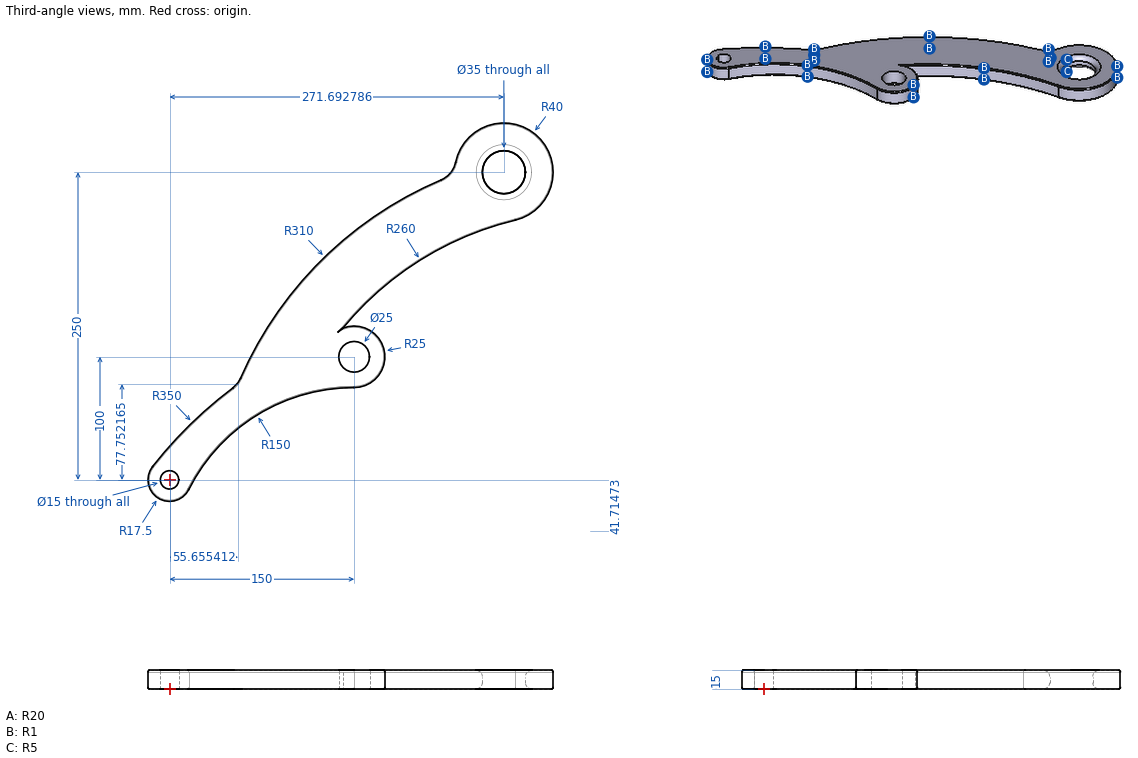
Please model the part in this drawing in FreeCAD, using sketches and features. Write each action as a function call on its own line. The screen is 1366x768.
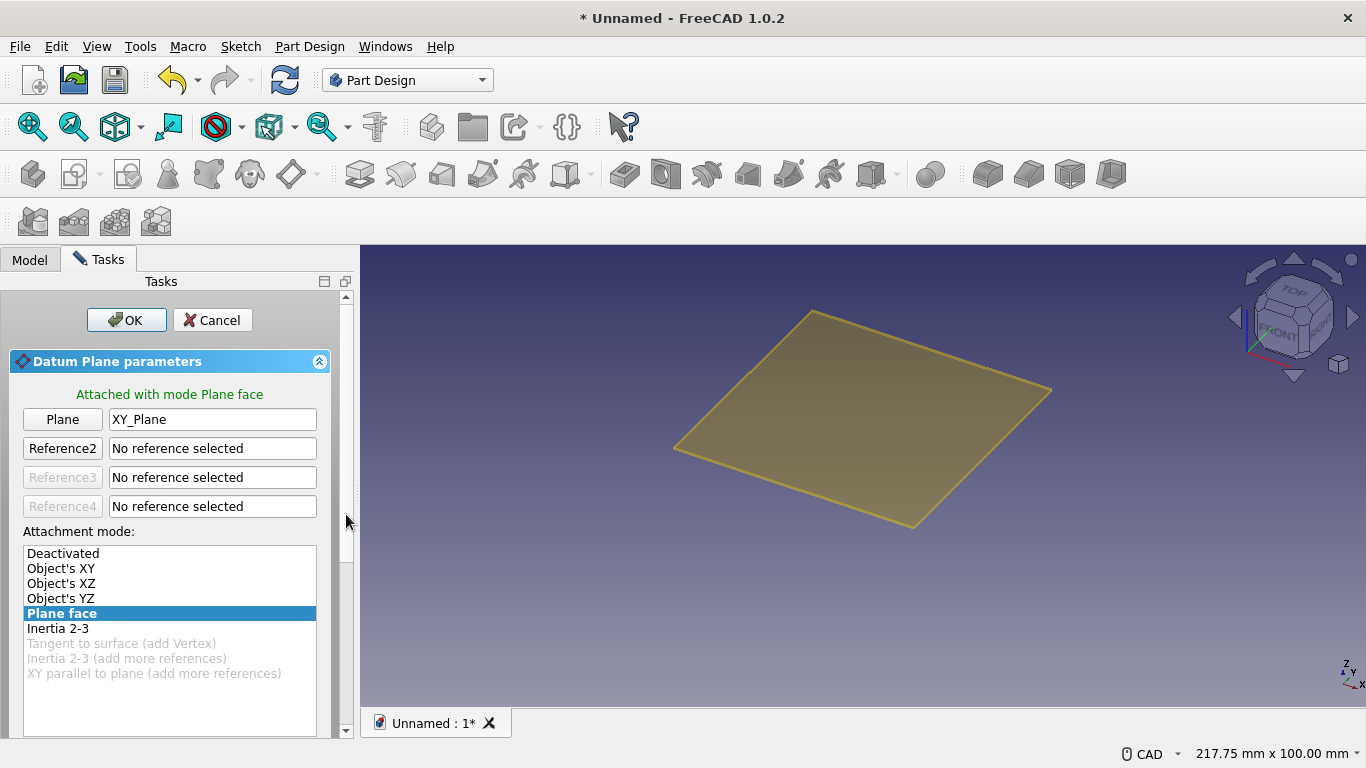
click(127, 320)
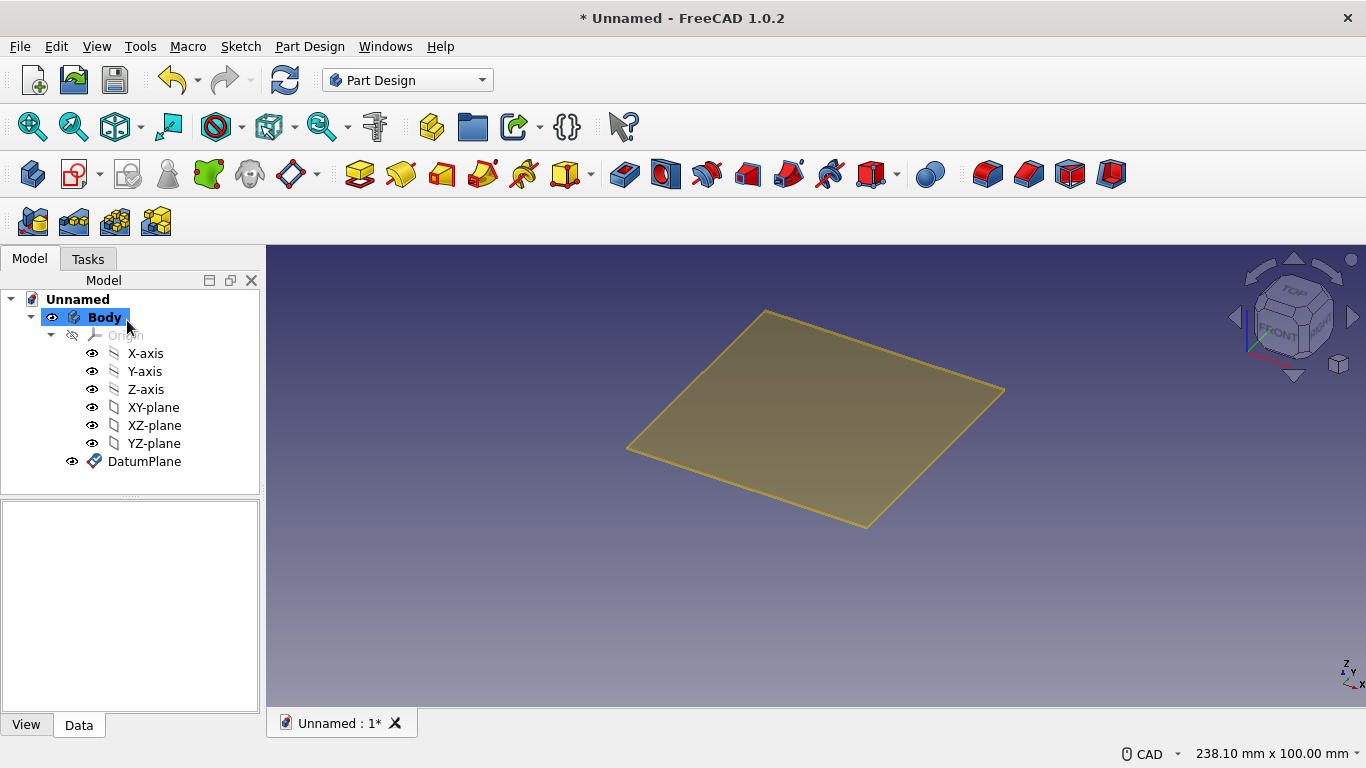
click(117, 461)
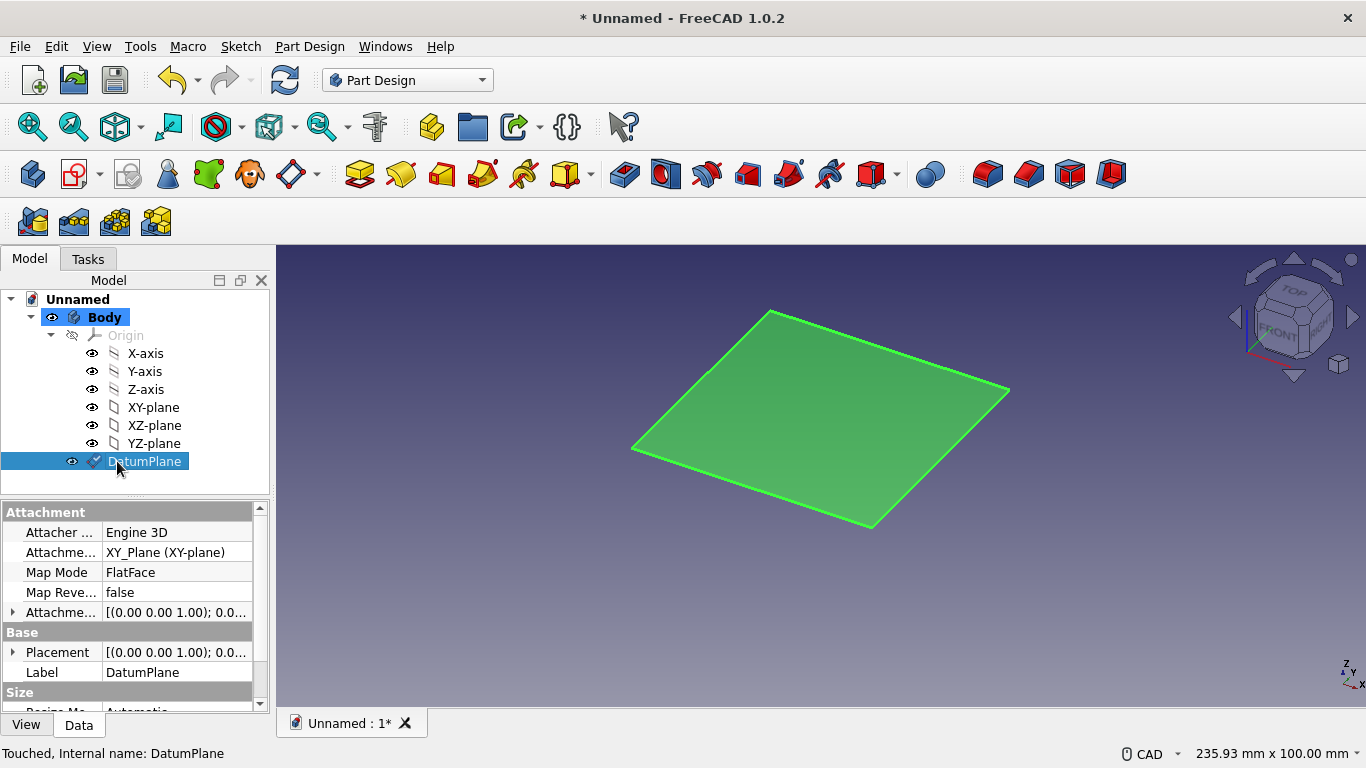
click(74, 174)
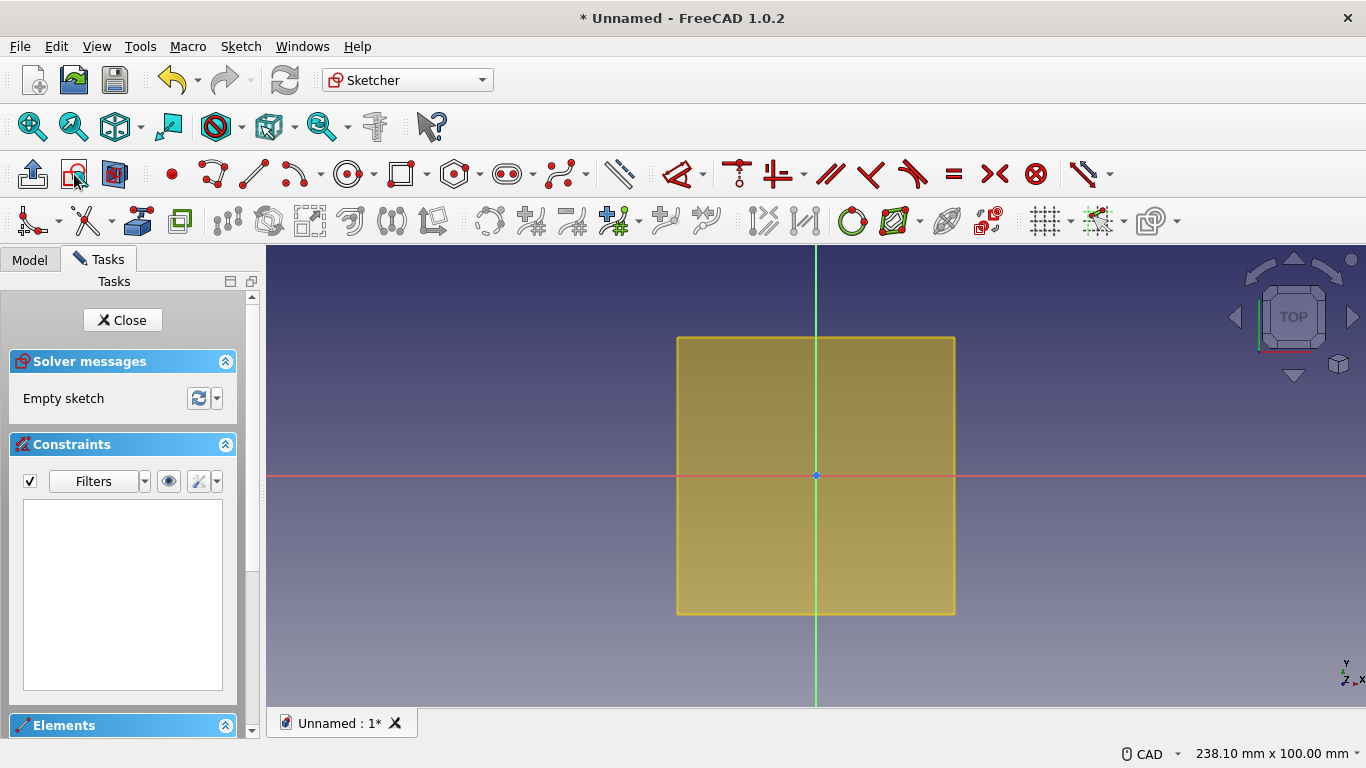
scroll(565, 632, down, 8)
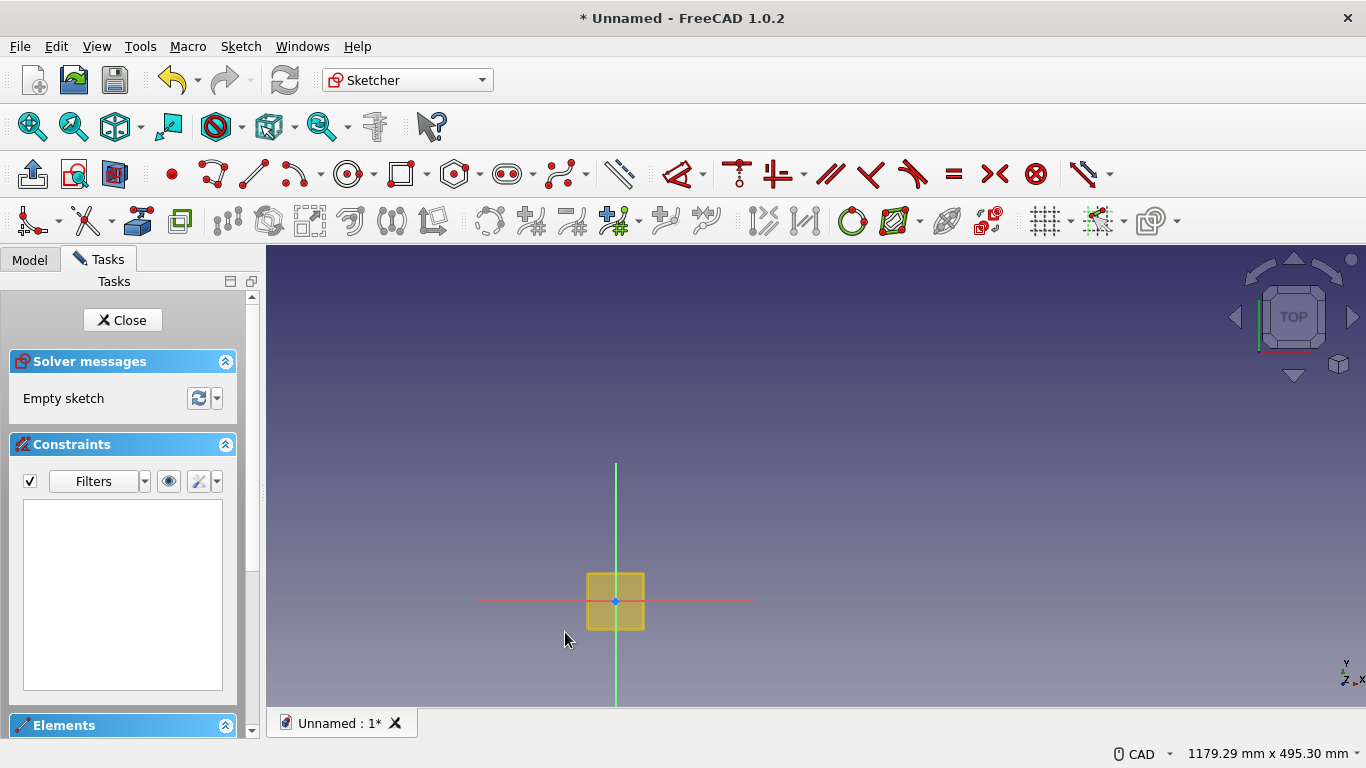
key(g)
key(3)
key(a)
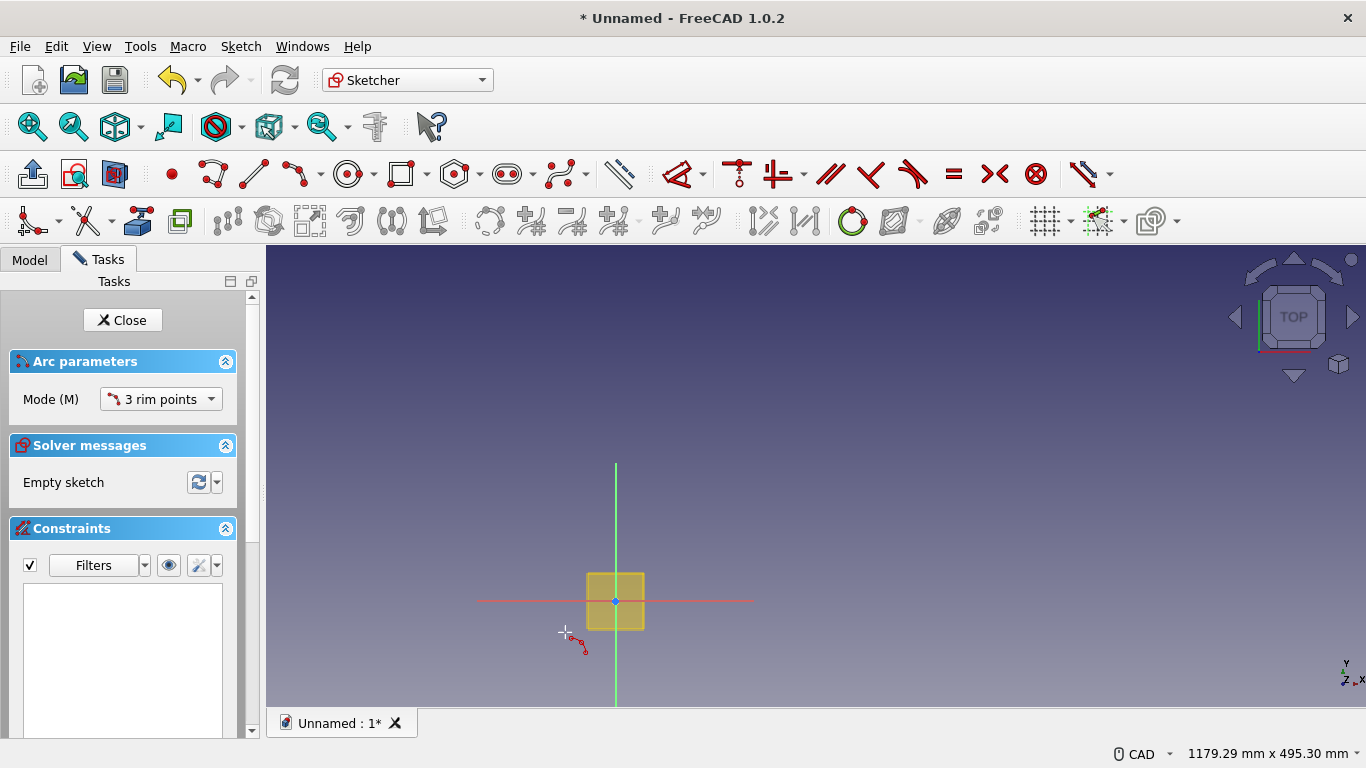
scroll(603, 591, up, 3)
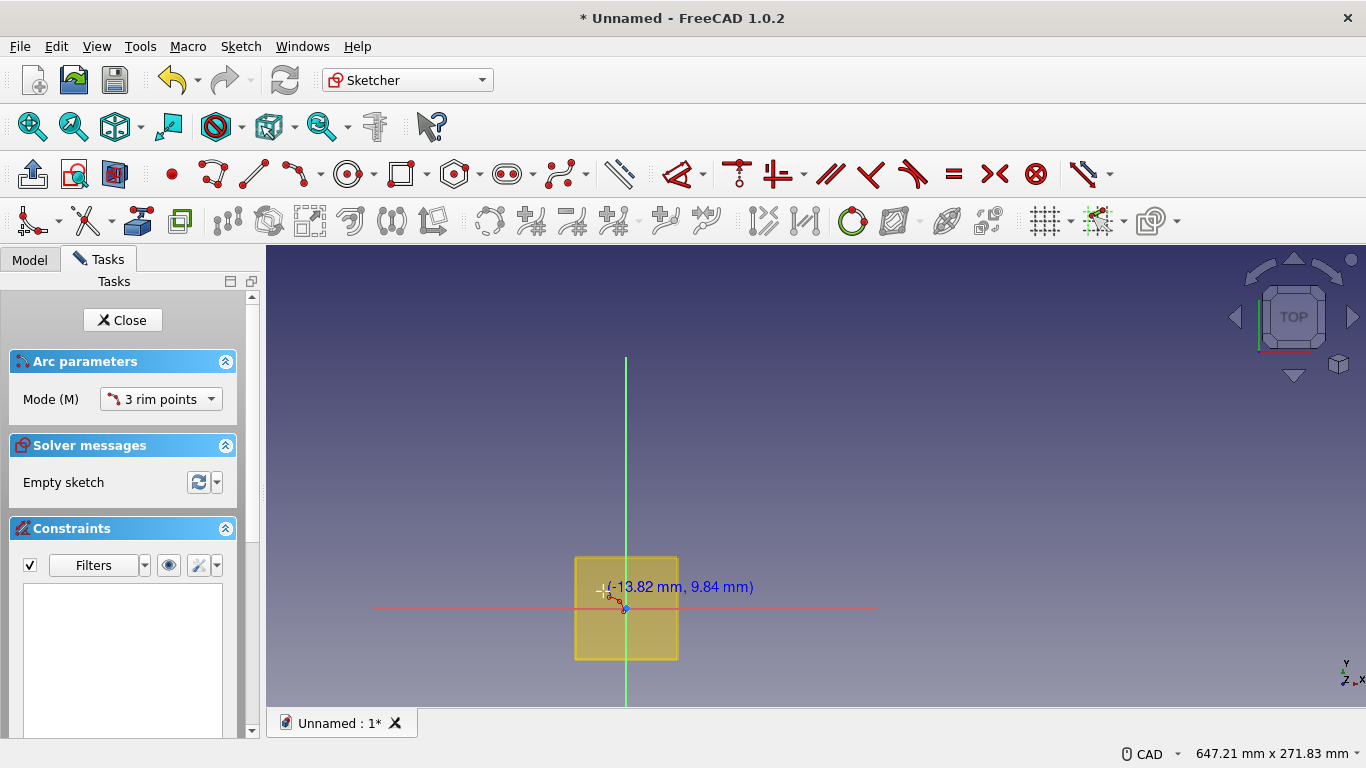
click(603, 591)
click(653, 622)
click(603, 627)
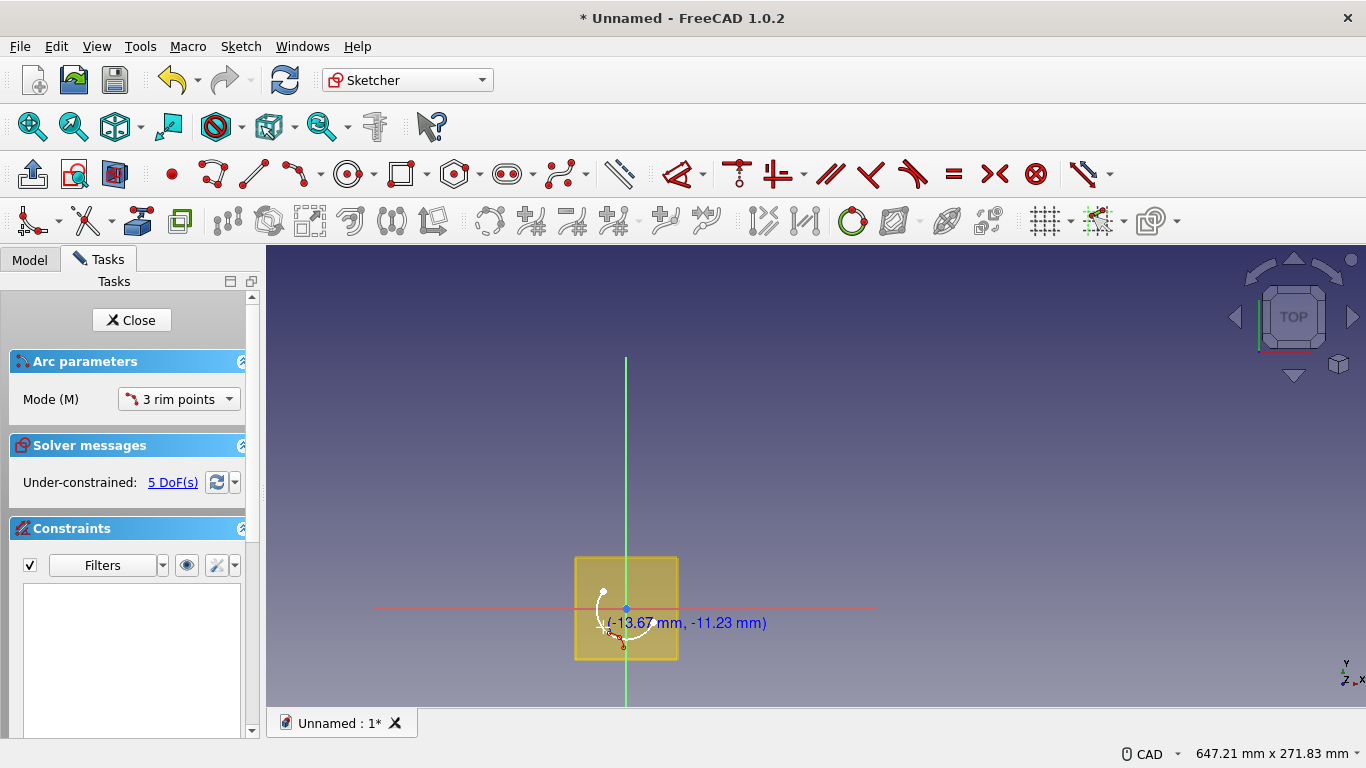
click(653, 623)
click(881, 481)
click(747, 519)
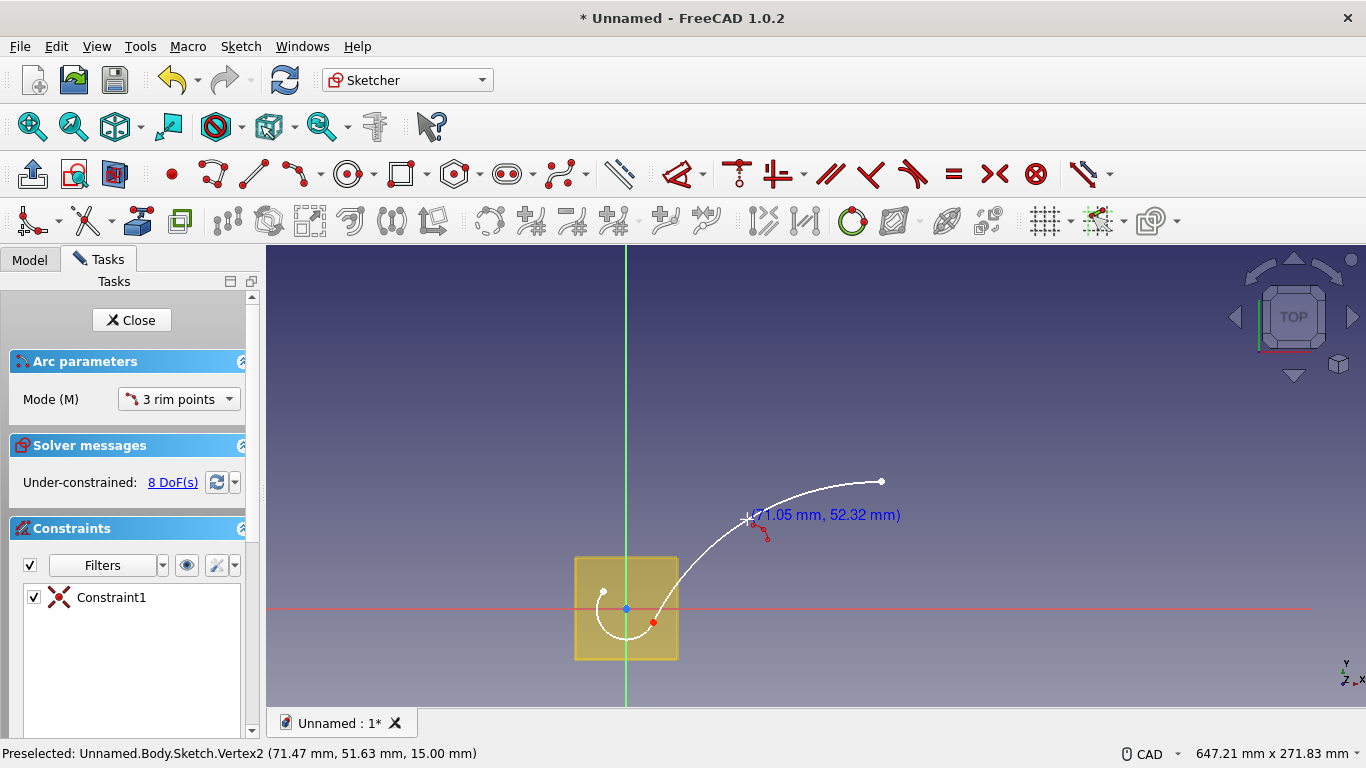
click(881, 482)
click(865, 400)
click(923, 431)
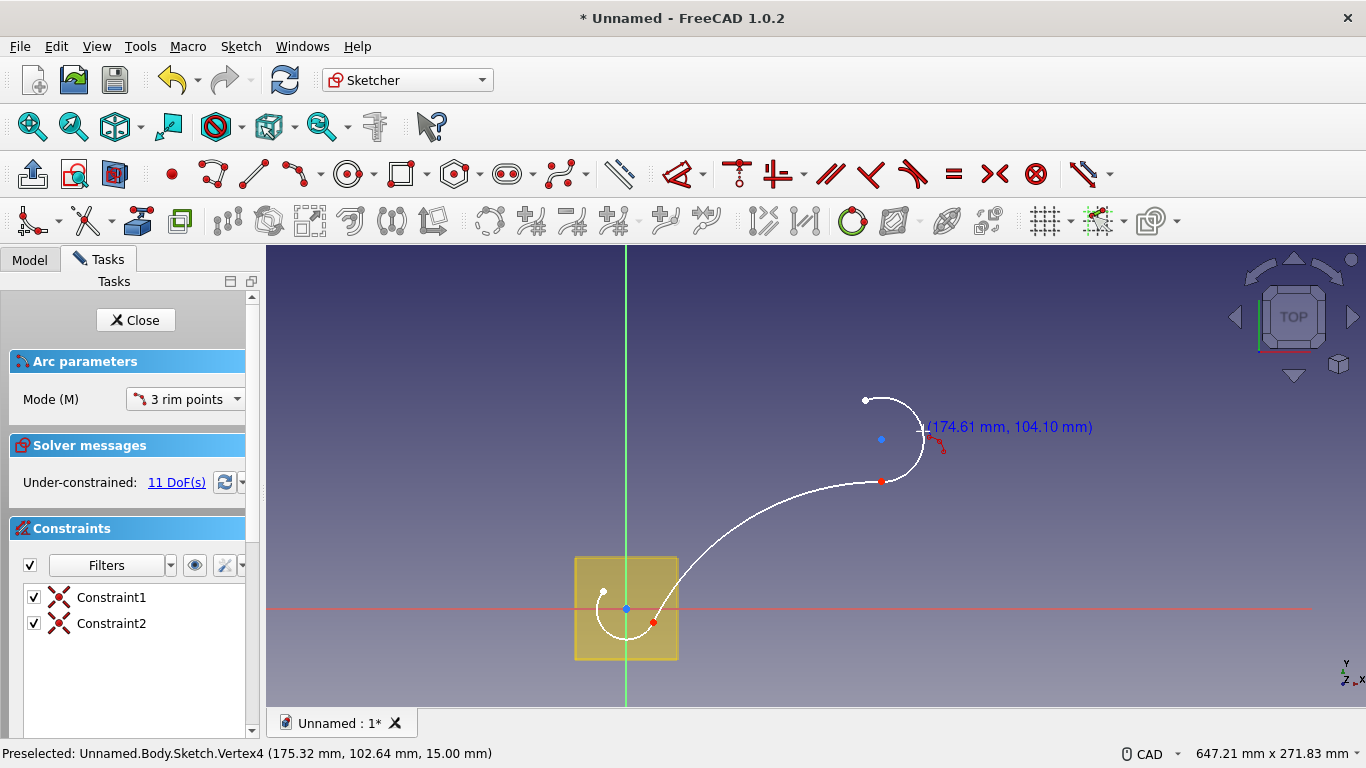
click(865, 401)